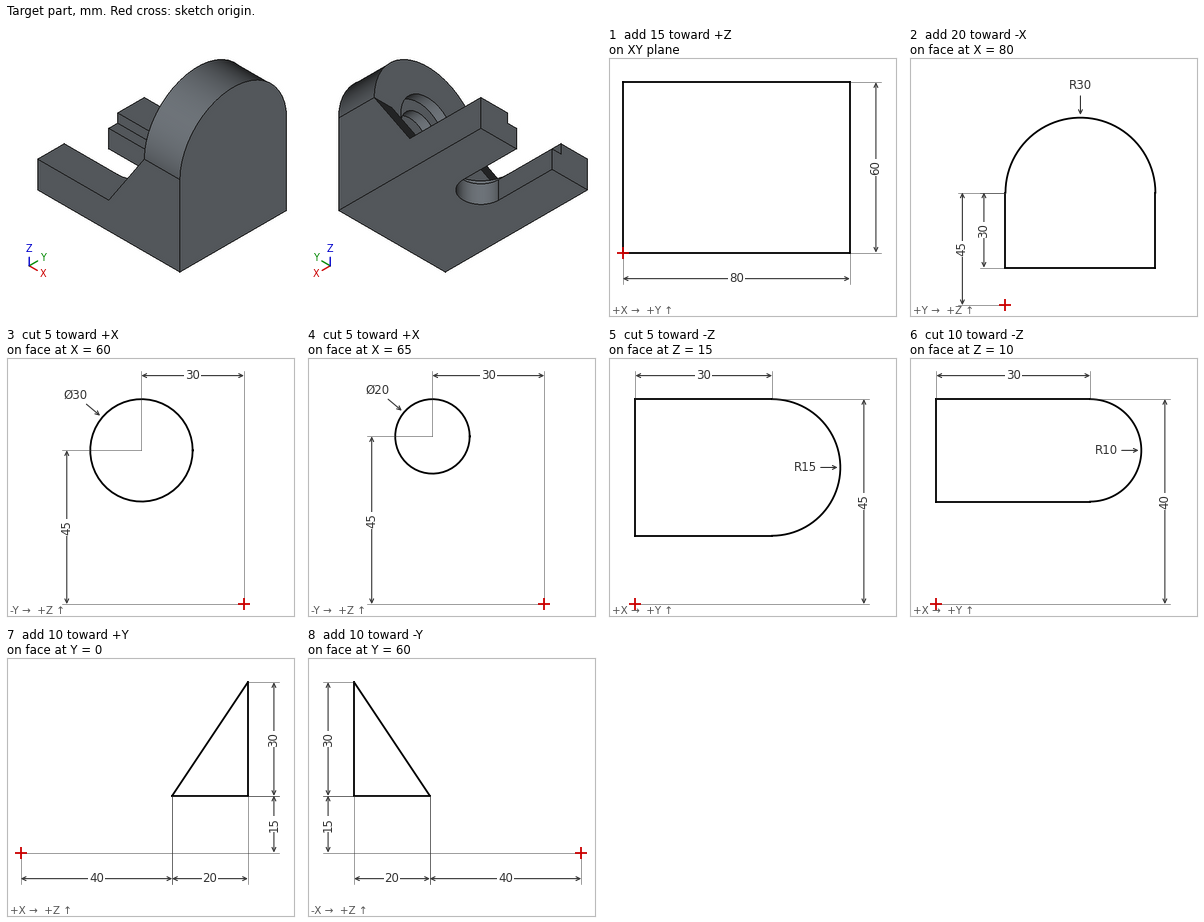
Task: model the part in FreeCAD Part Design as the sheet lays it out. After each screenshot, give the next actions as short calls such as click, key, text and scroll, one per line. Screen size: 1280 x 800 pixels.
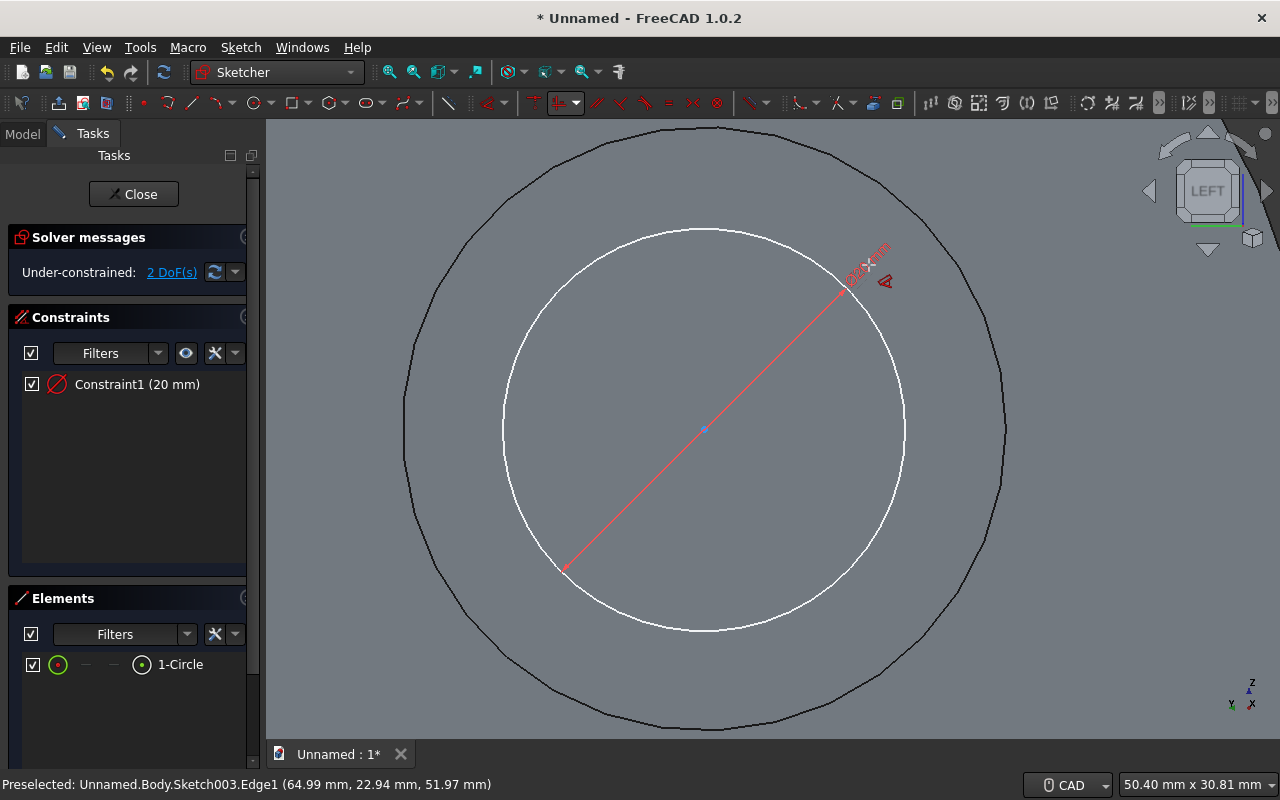
click(704, 430)
click(815, 396)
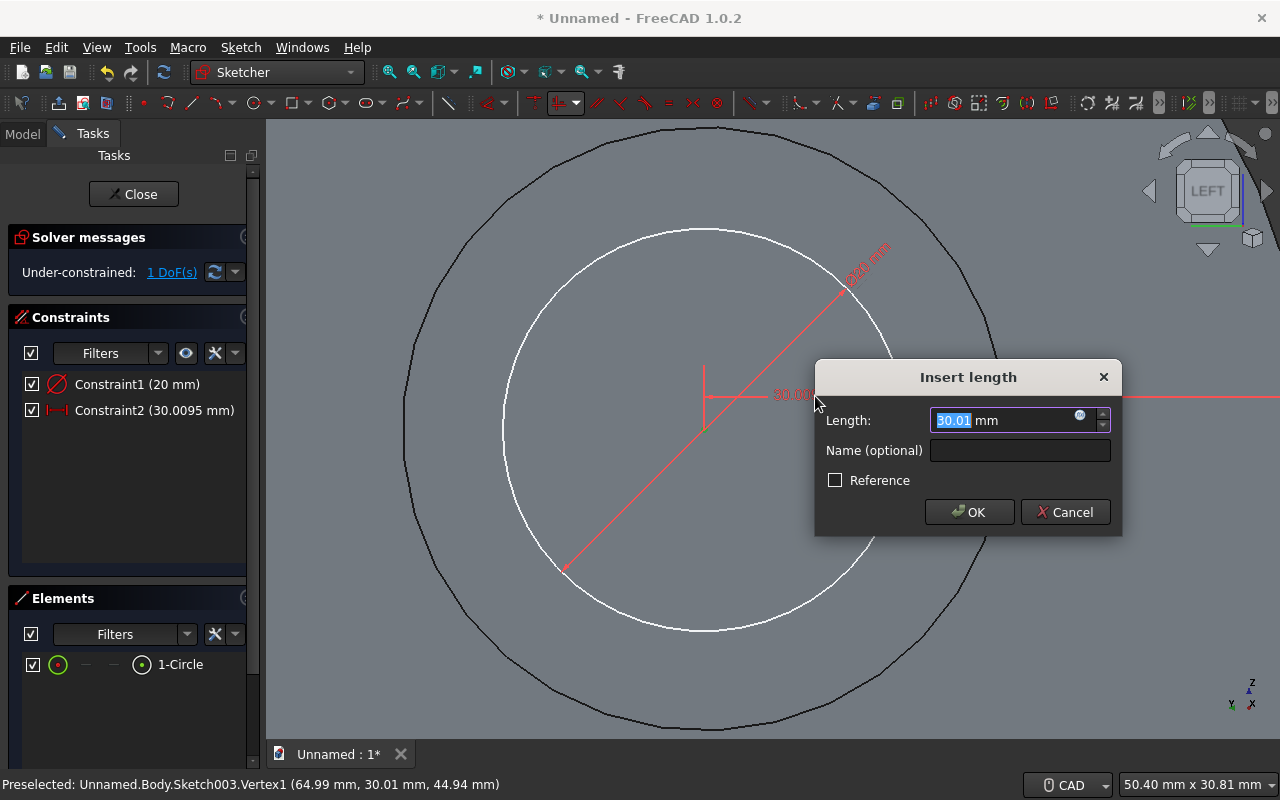
text(30)
key(Return)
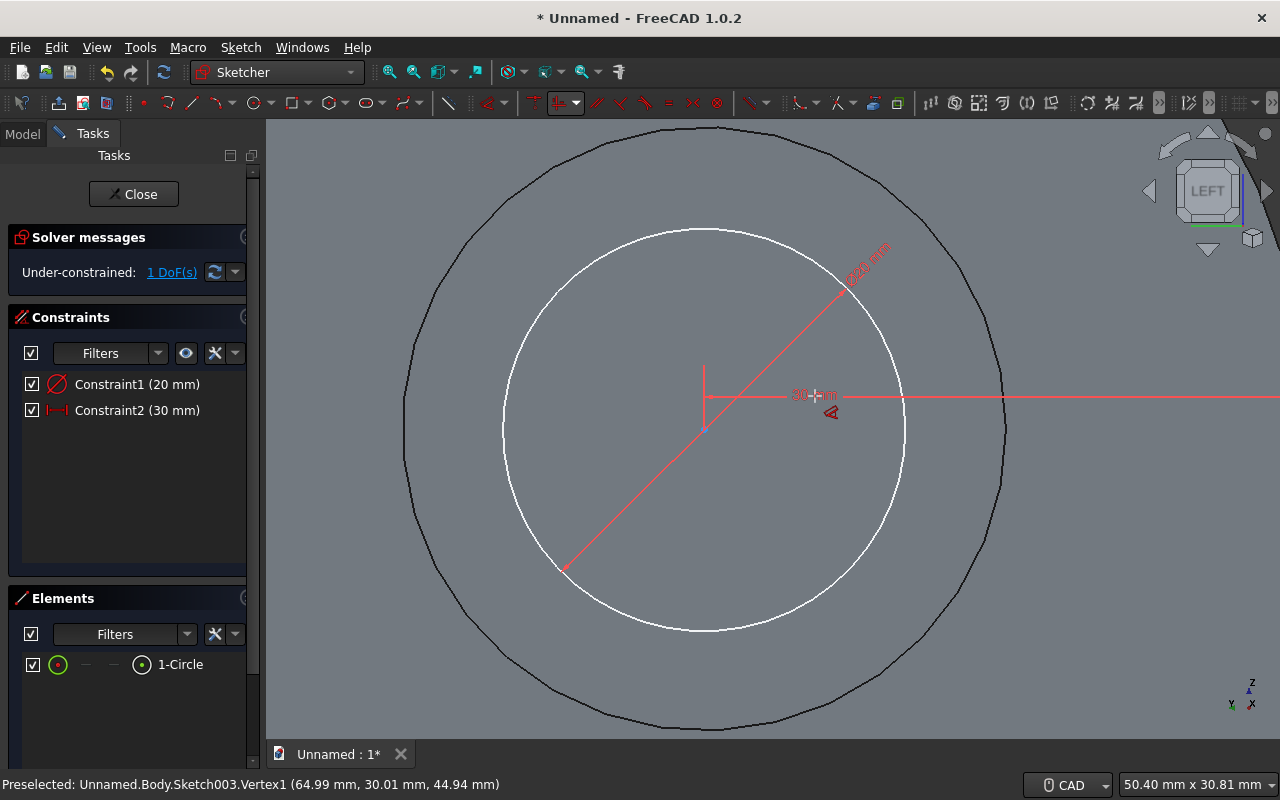
click(704, 430)
click(670, 571)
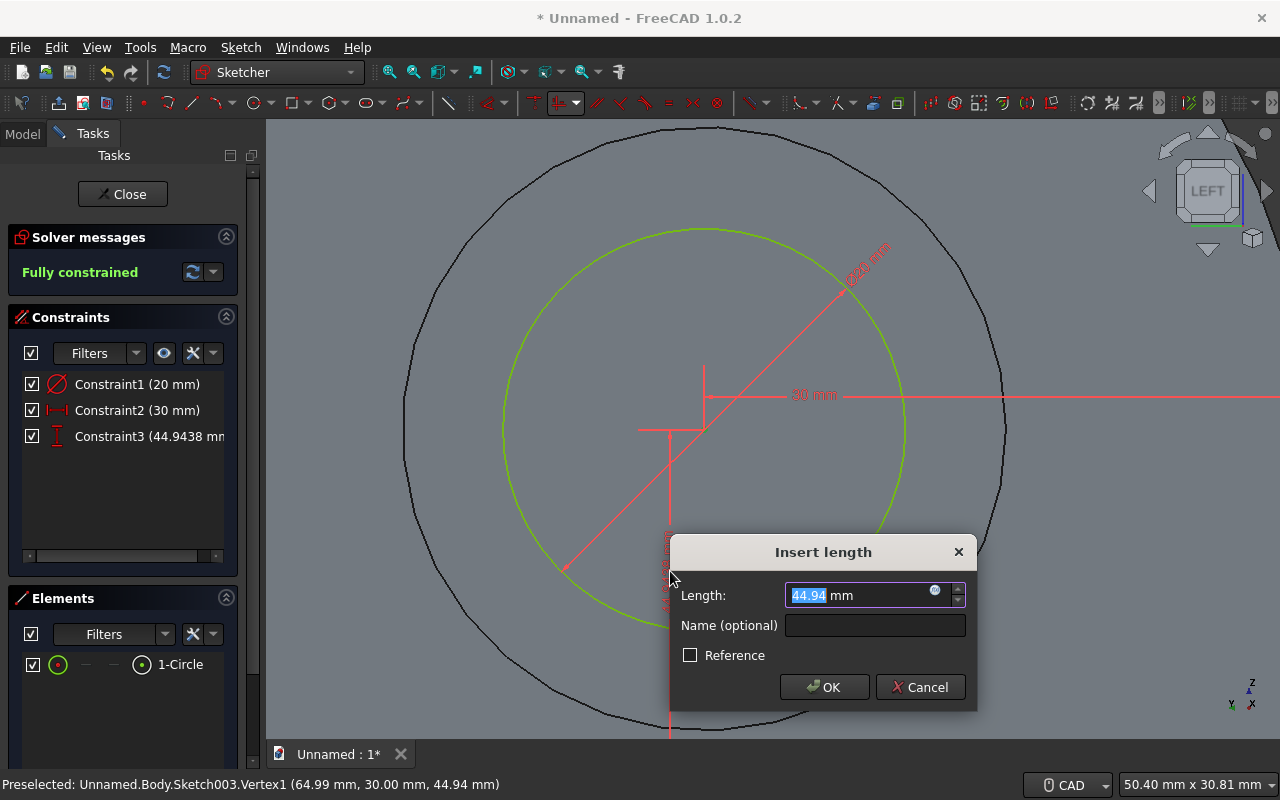
text(45)
key(Return)
key(Escape)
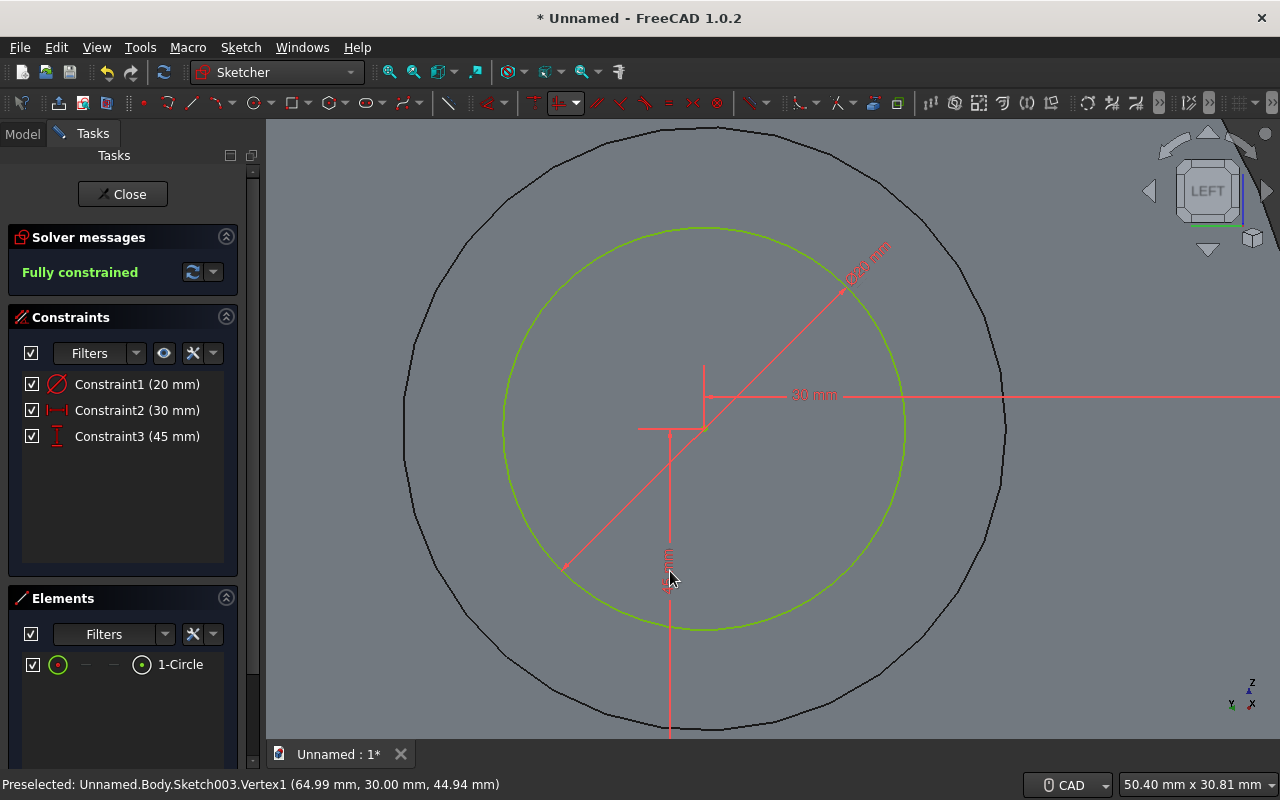
click(123, 194)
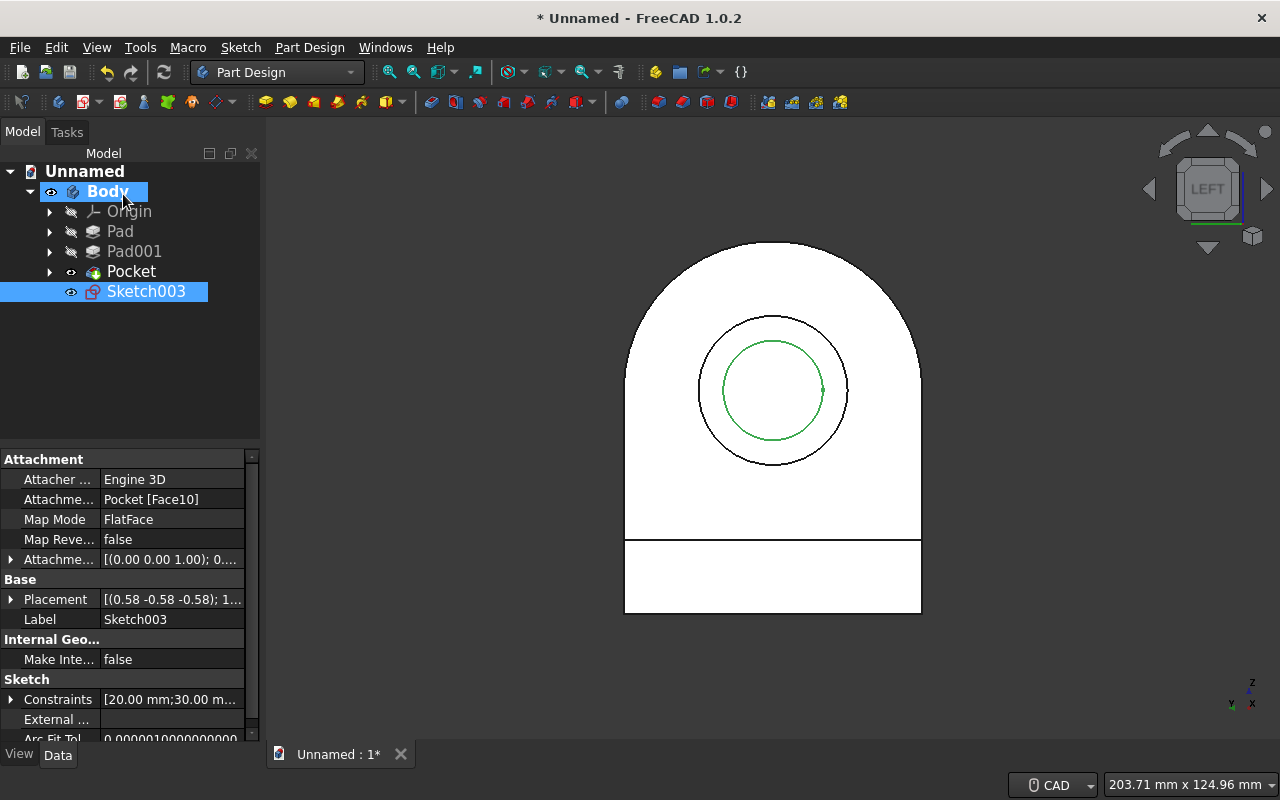
click(432, 102)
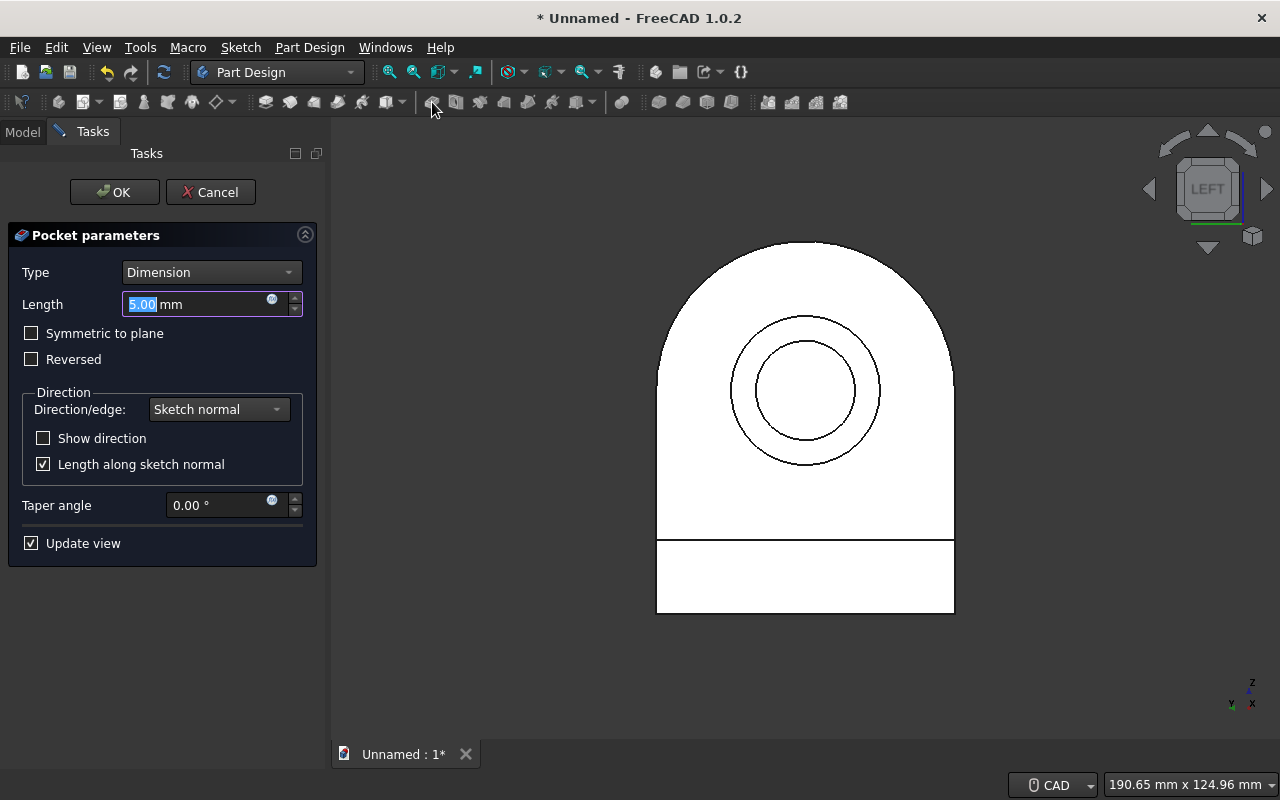
text(5)
key(Tab)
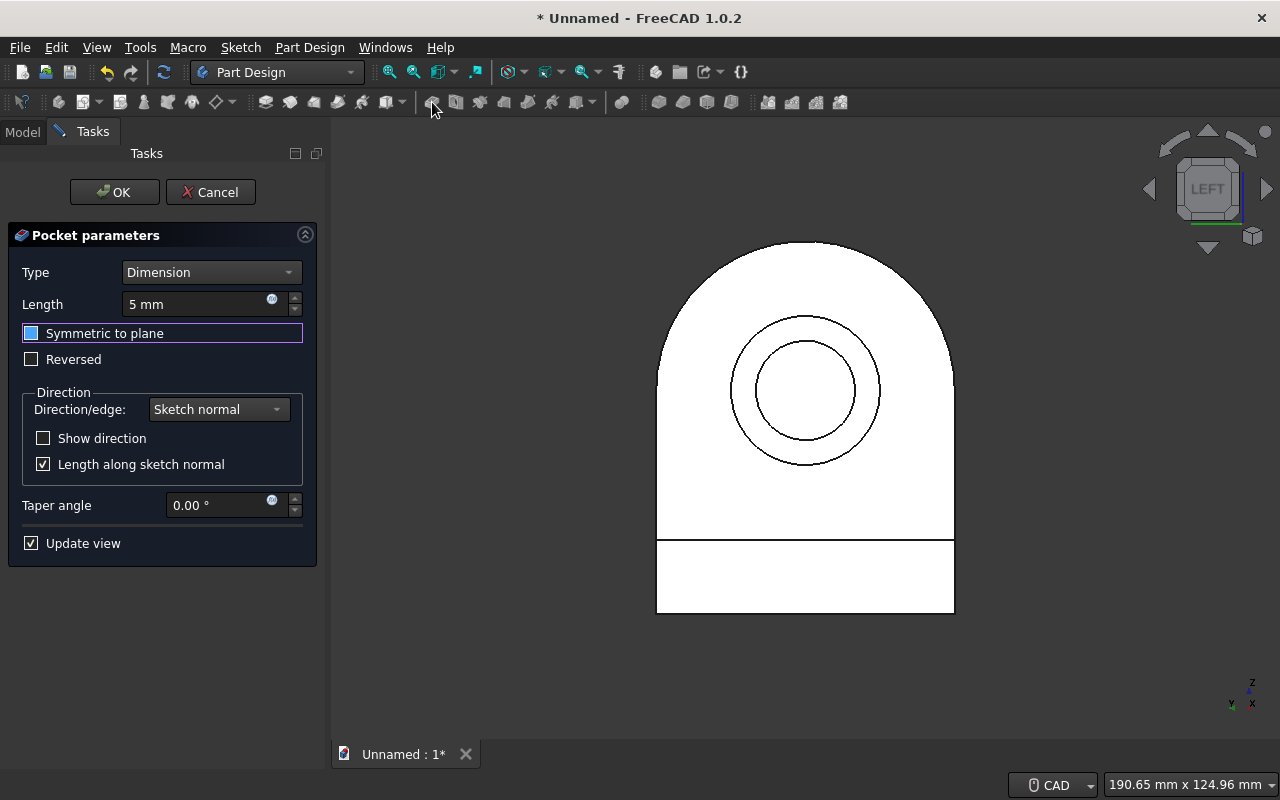
click(115, 192)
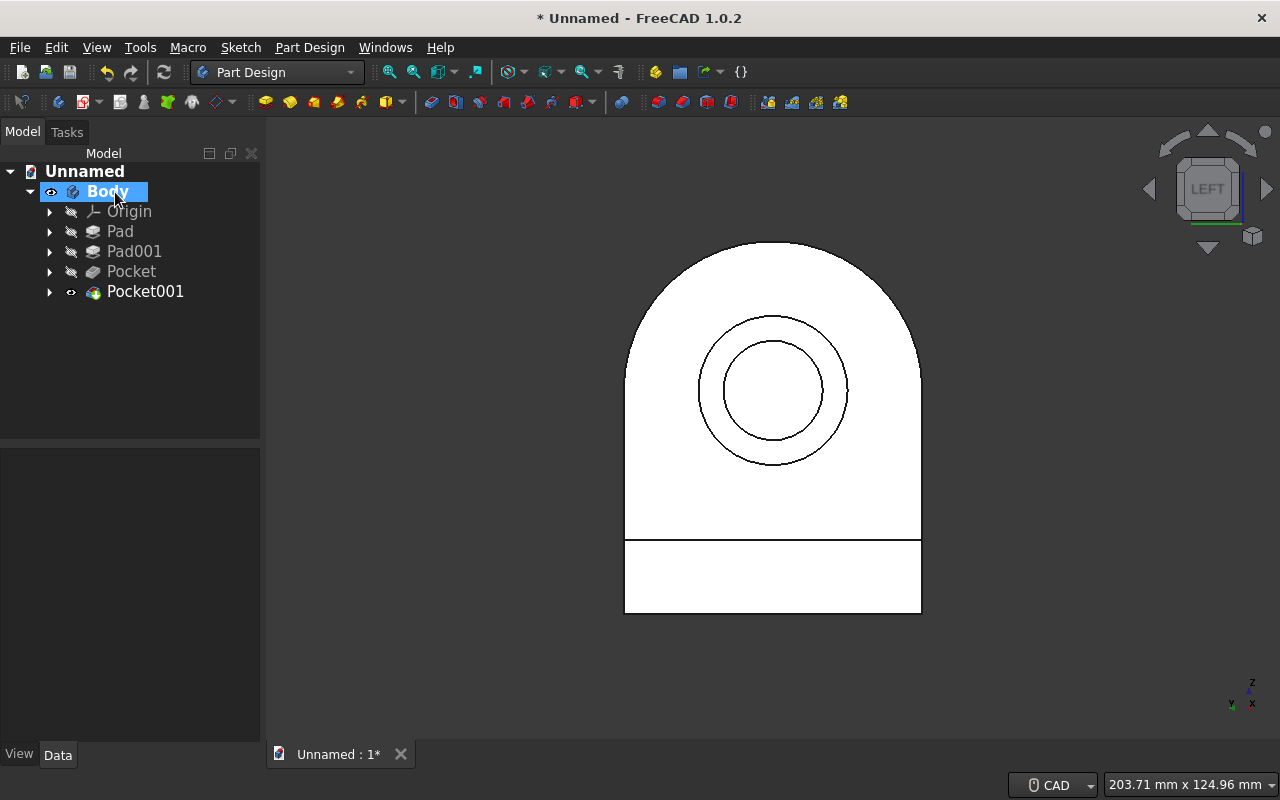
key(0)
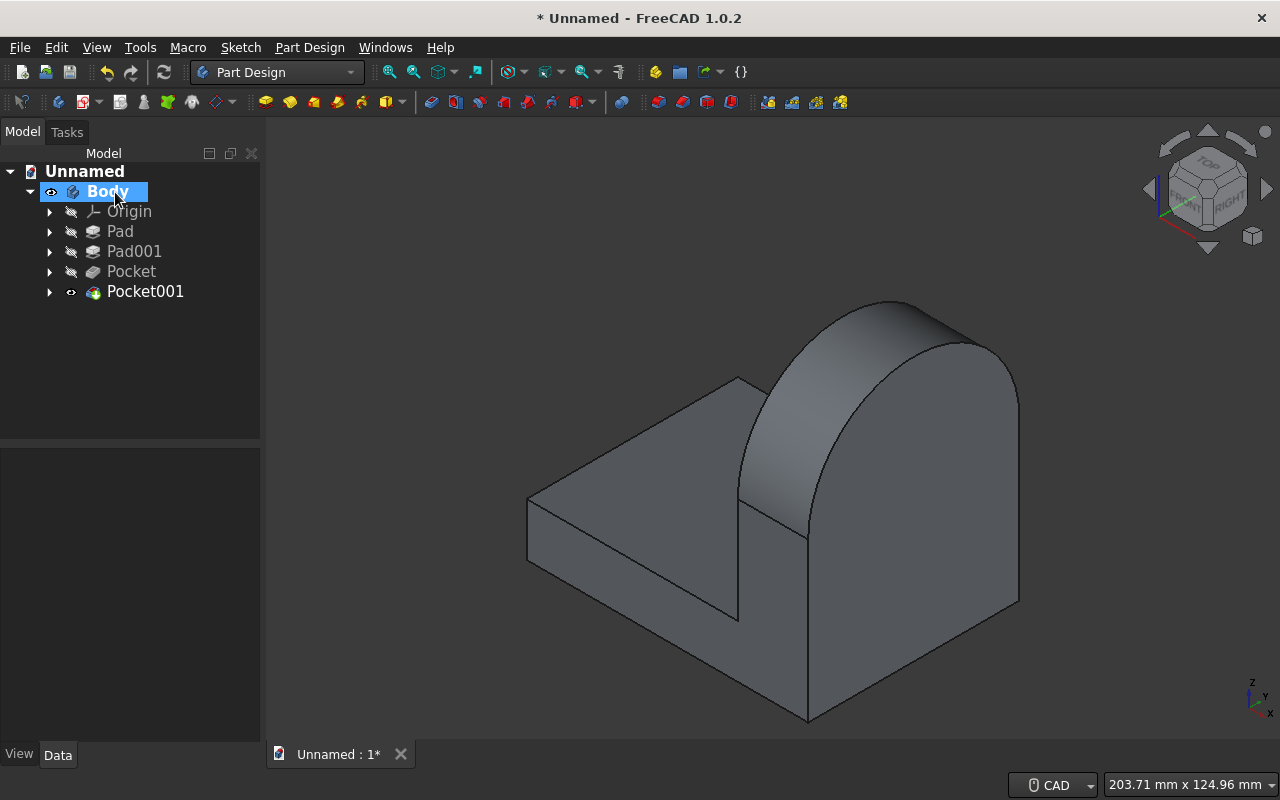
click(708, 515)